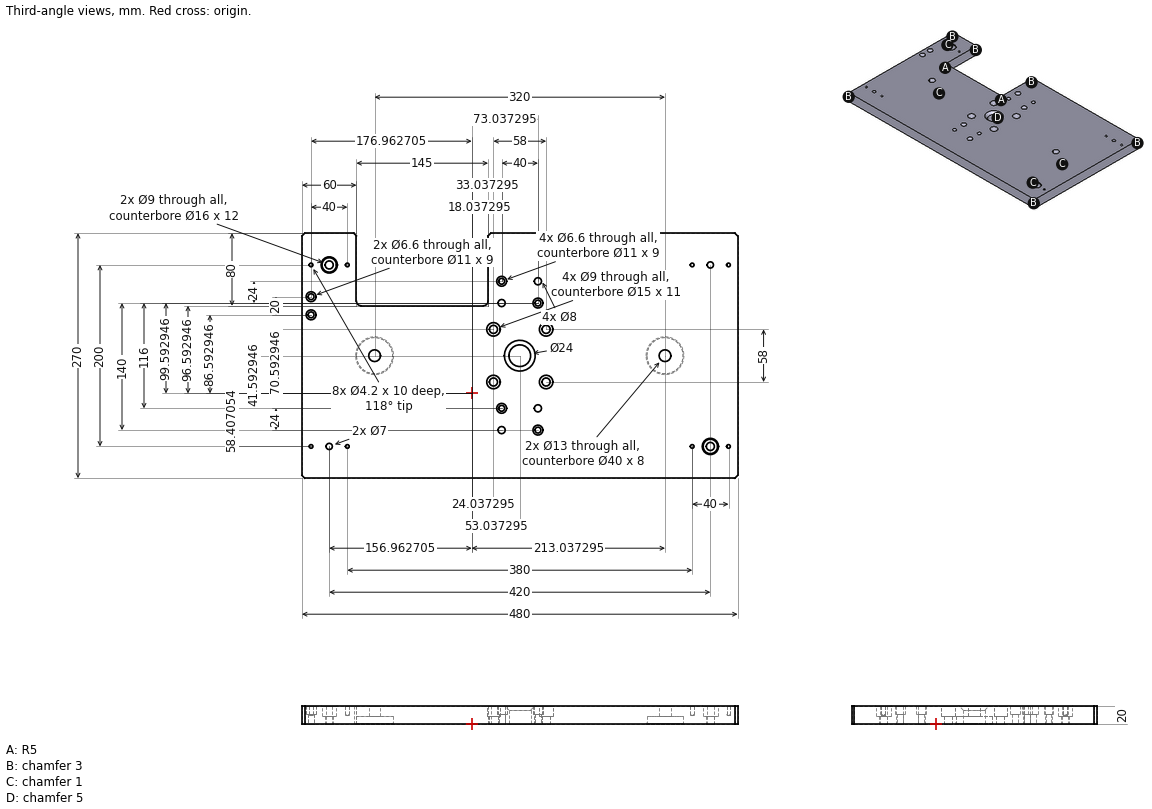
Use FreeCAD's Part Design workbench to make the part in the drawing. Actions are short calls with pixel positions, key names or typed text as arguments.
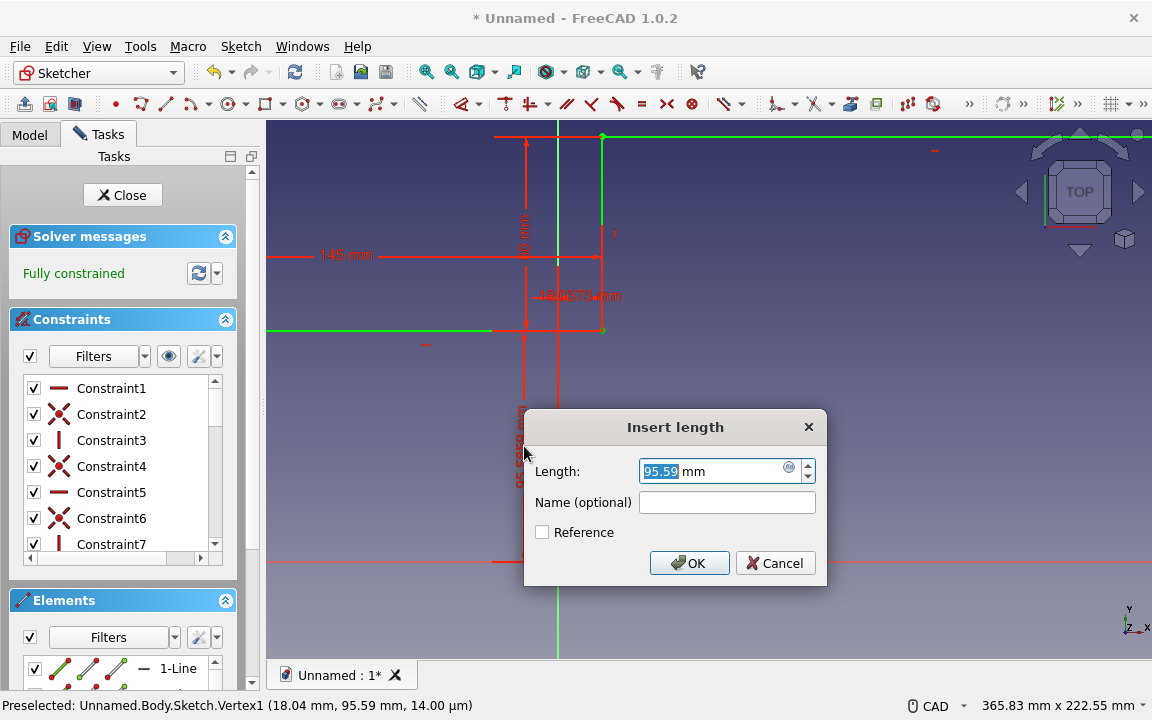
text(96.592946)
key(Return)
key(Escape)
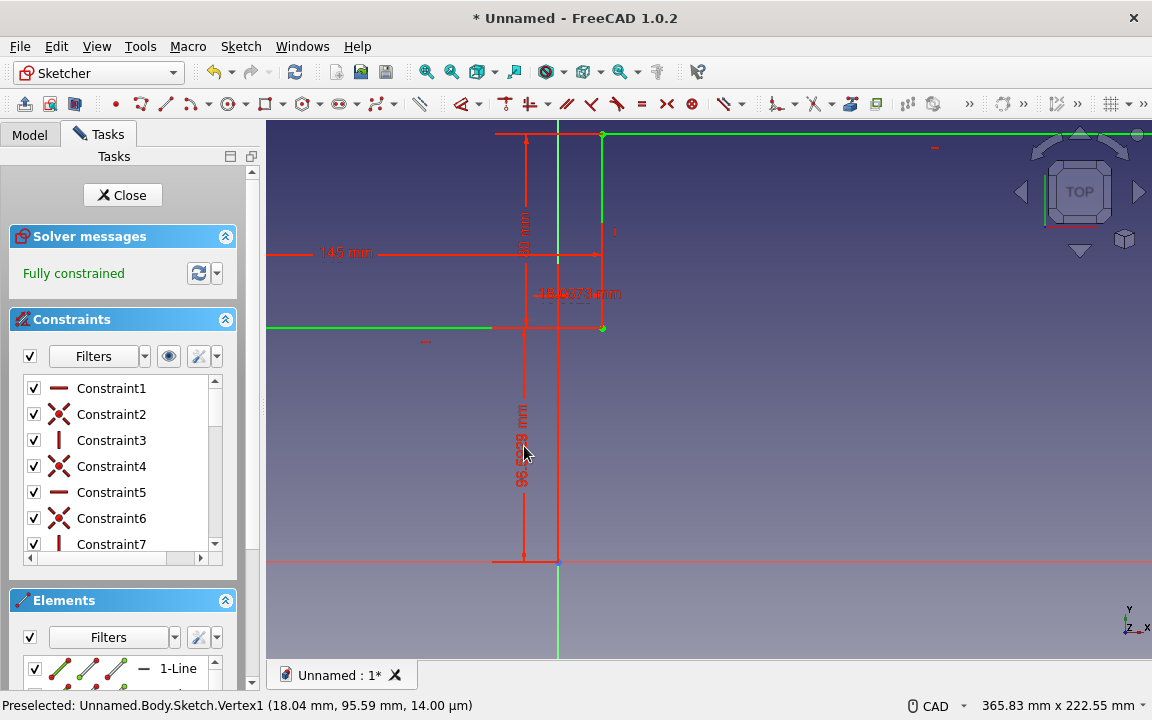
click(123, 195)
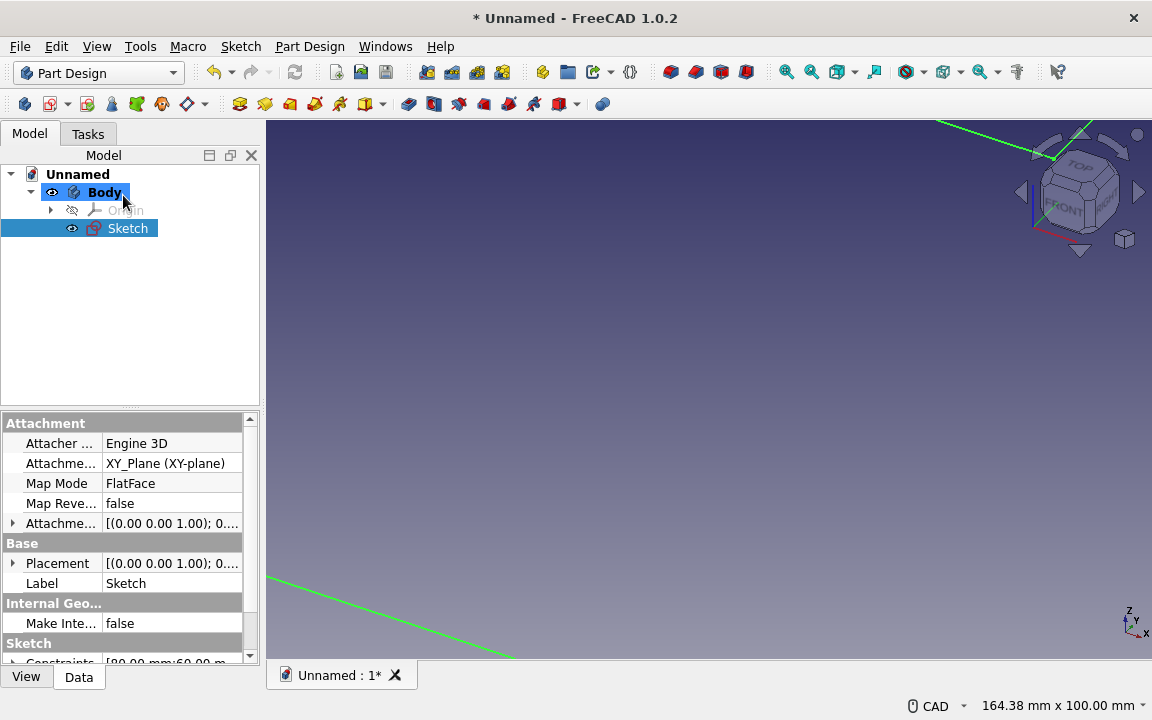
click(240, 104)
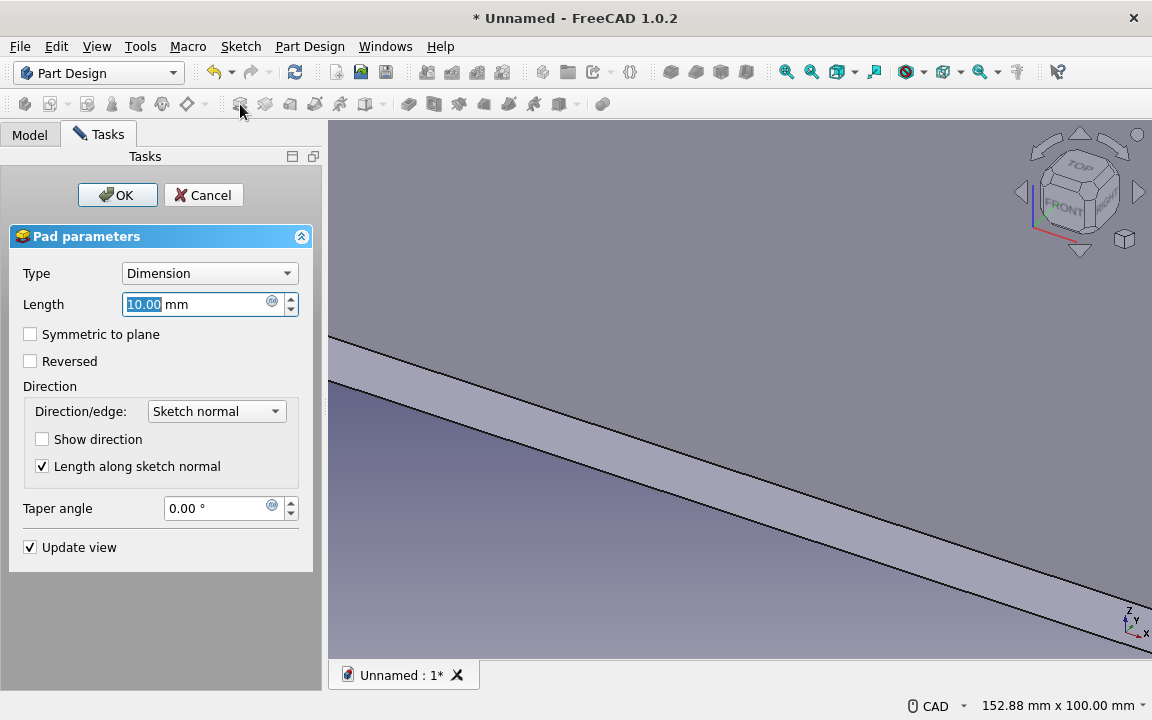
text(20)
key(Tab)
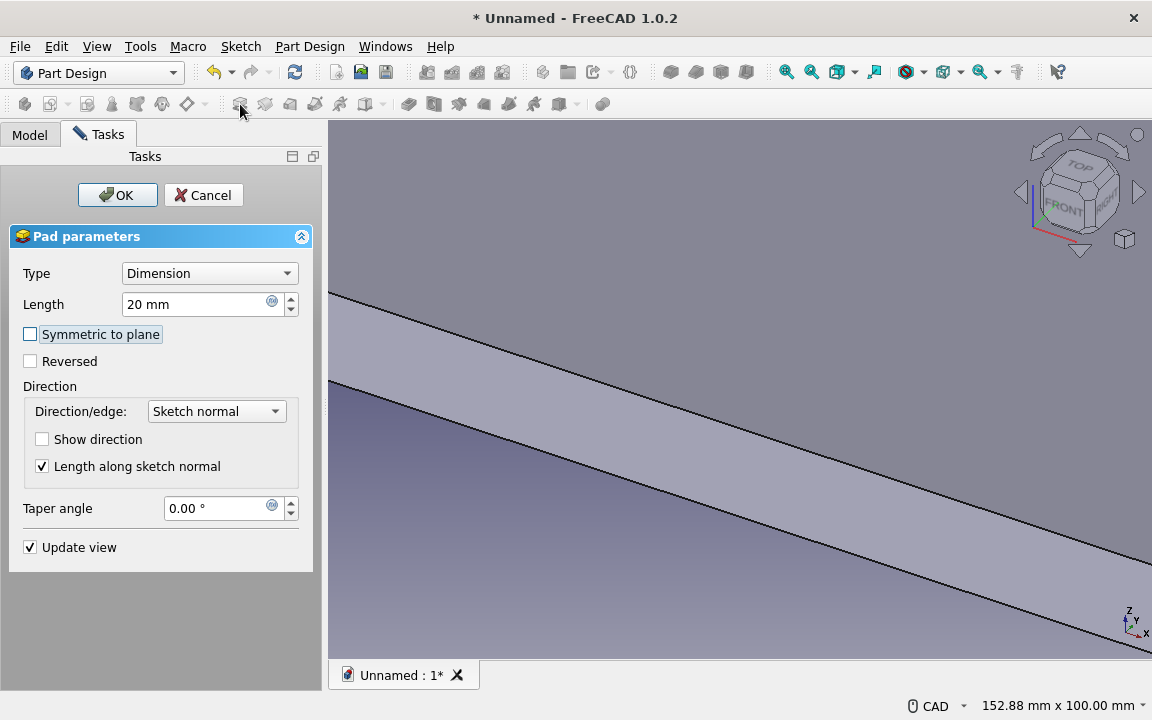
click(118, 195)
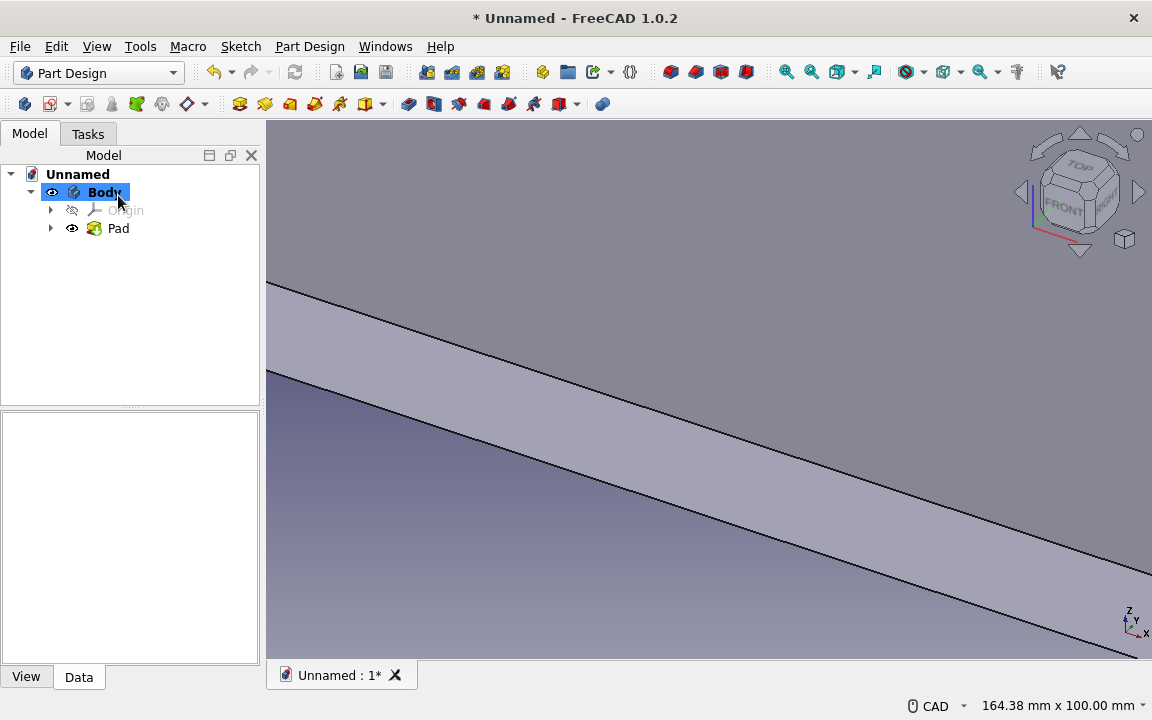
click(787, 72)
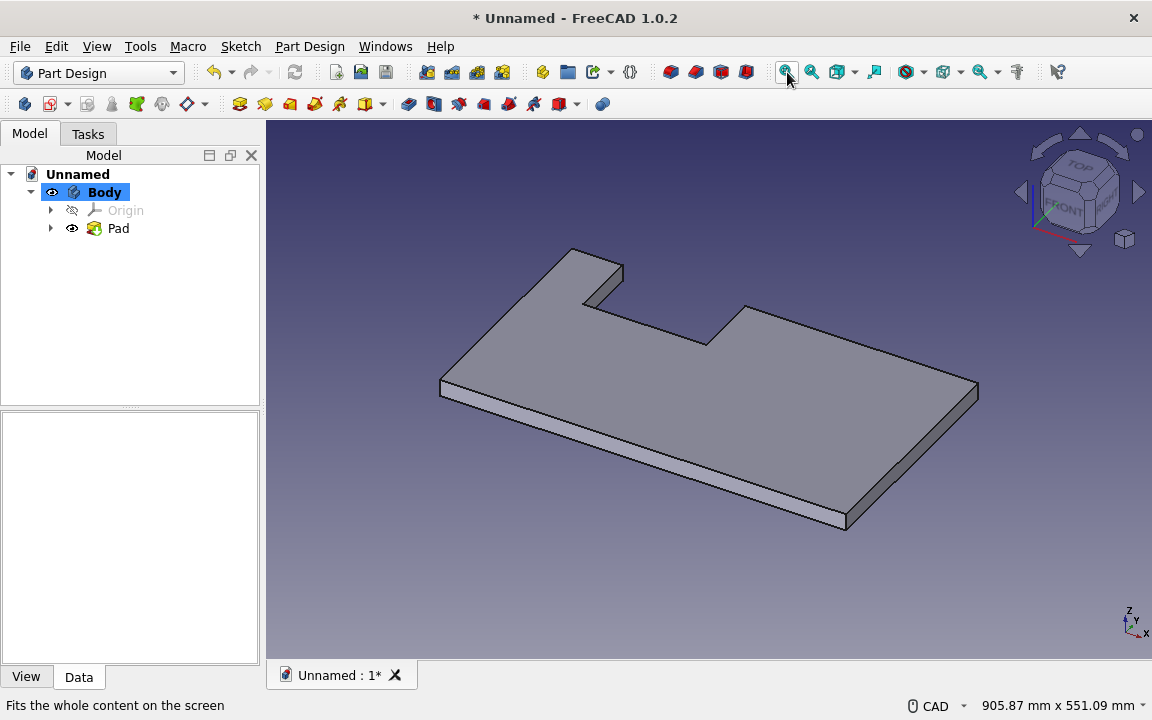
scroll(583, 311, up, 4)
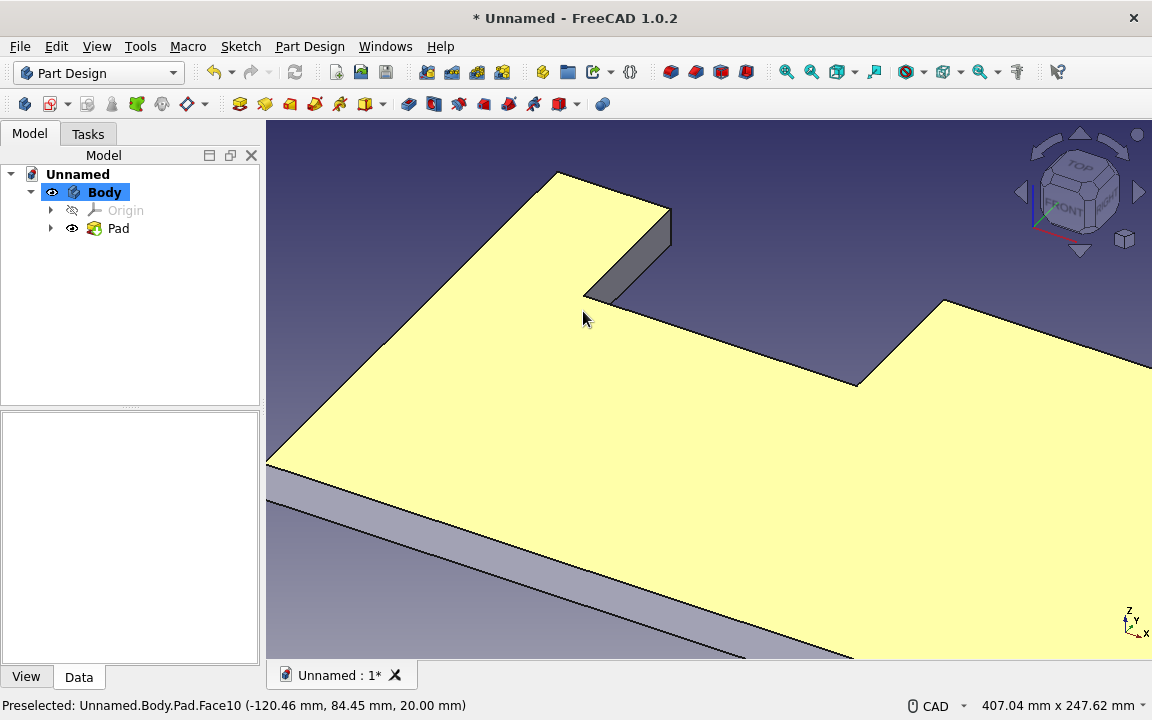
key(v)
key(f)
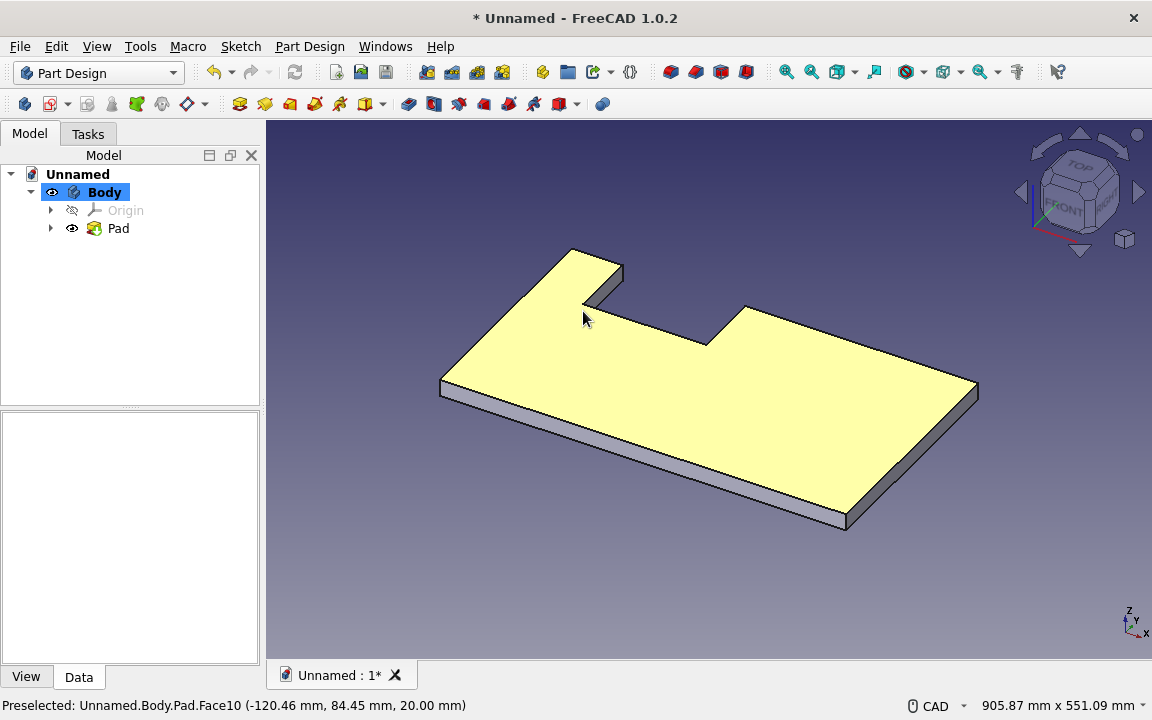
key(0)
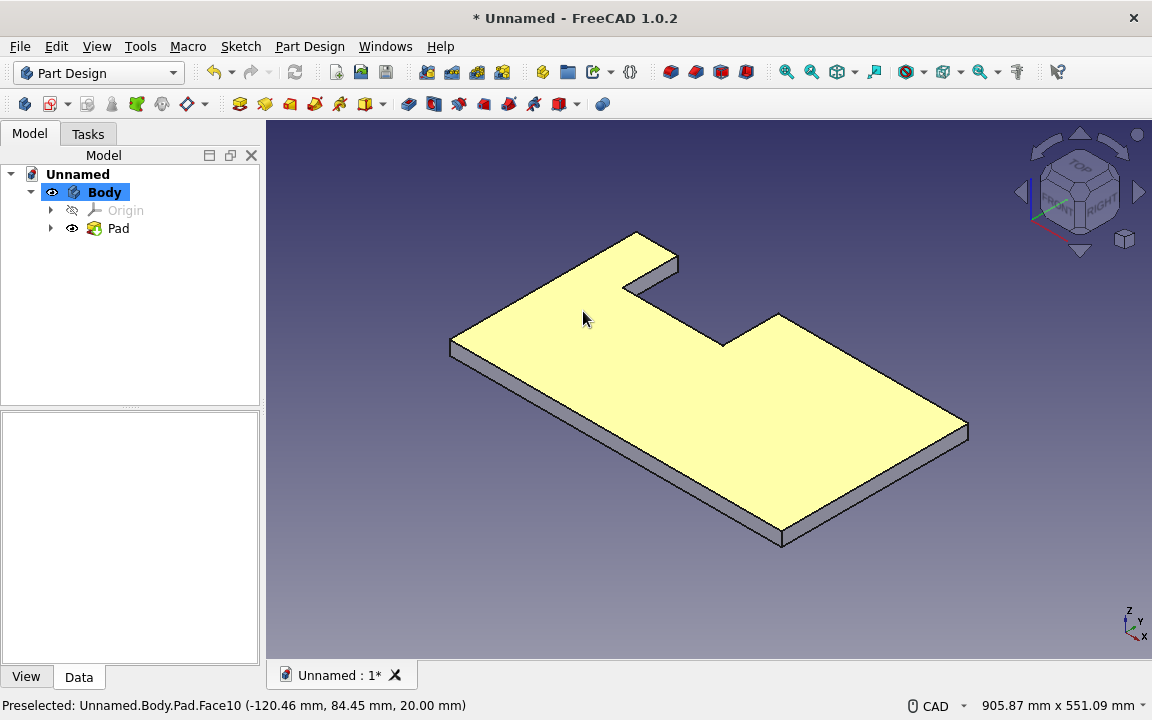
scroll(623, 295, up, 4)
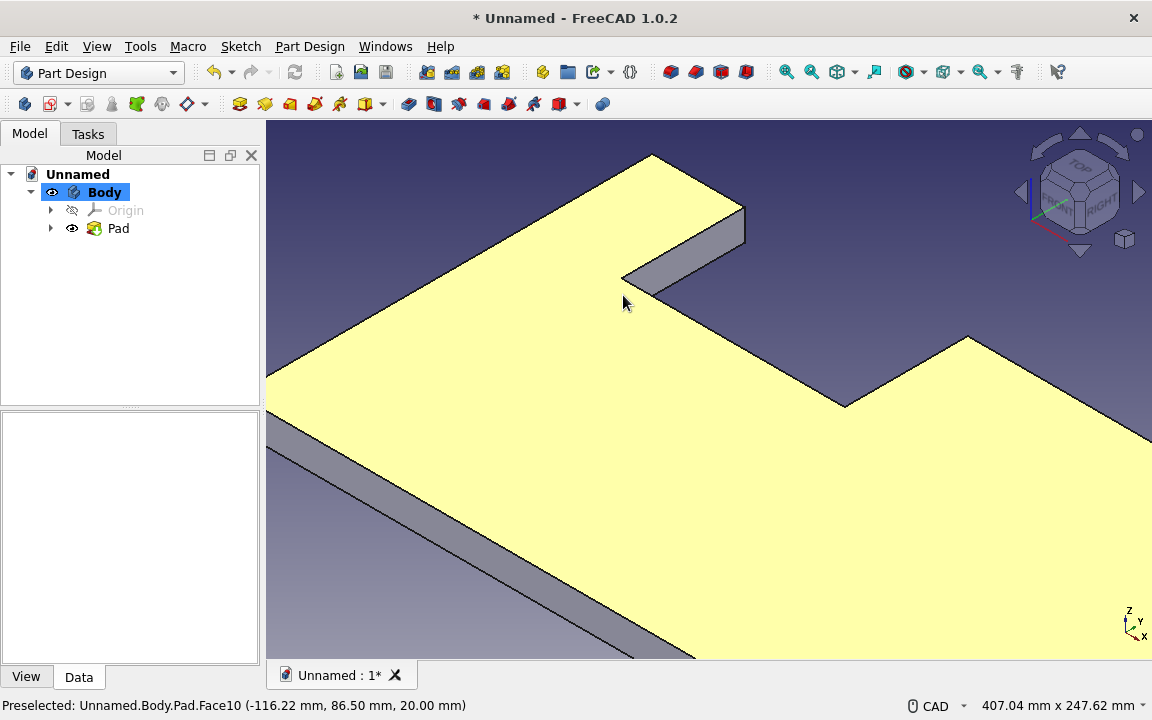
key(v)
key(f)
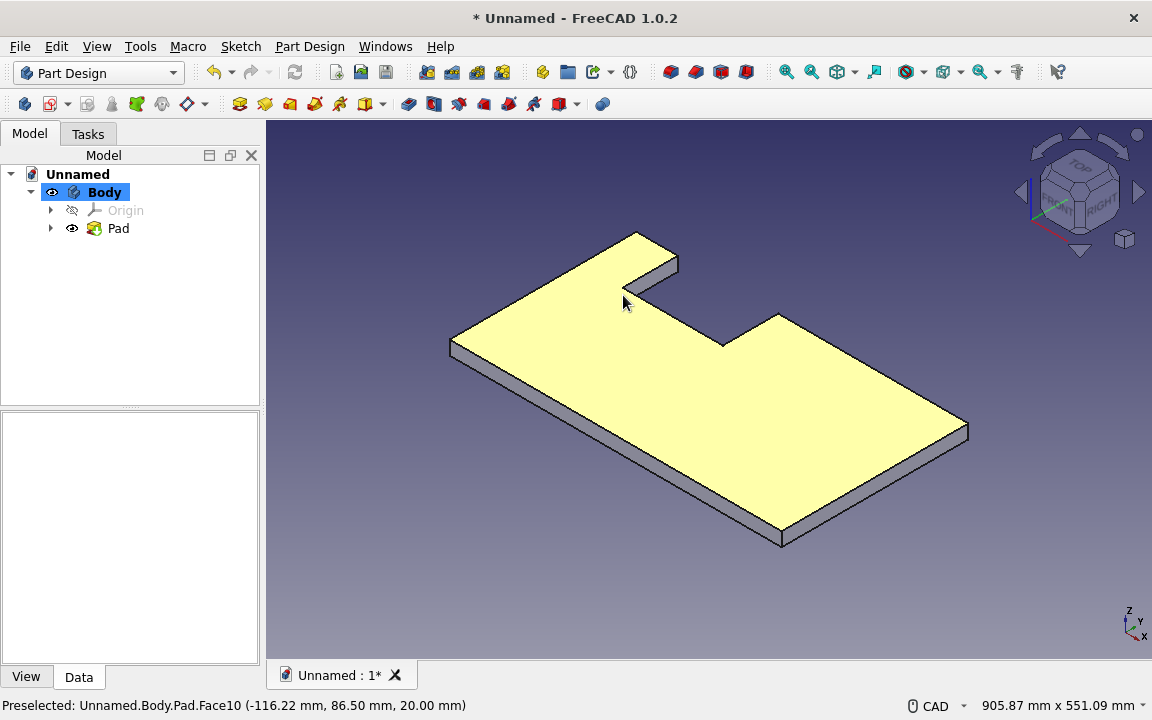
key(2)